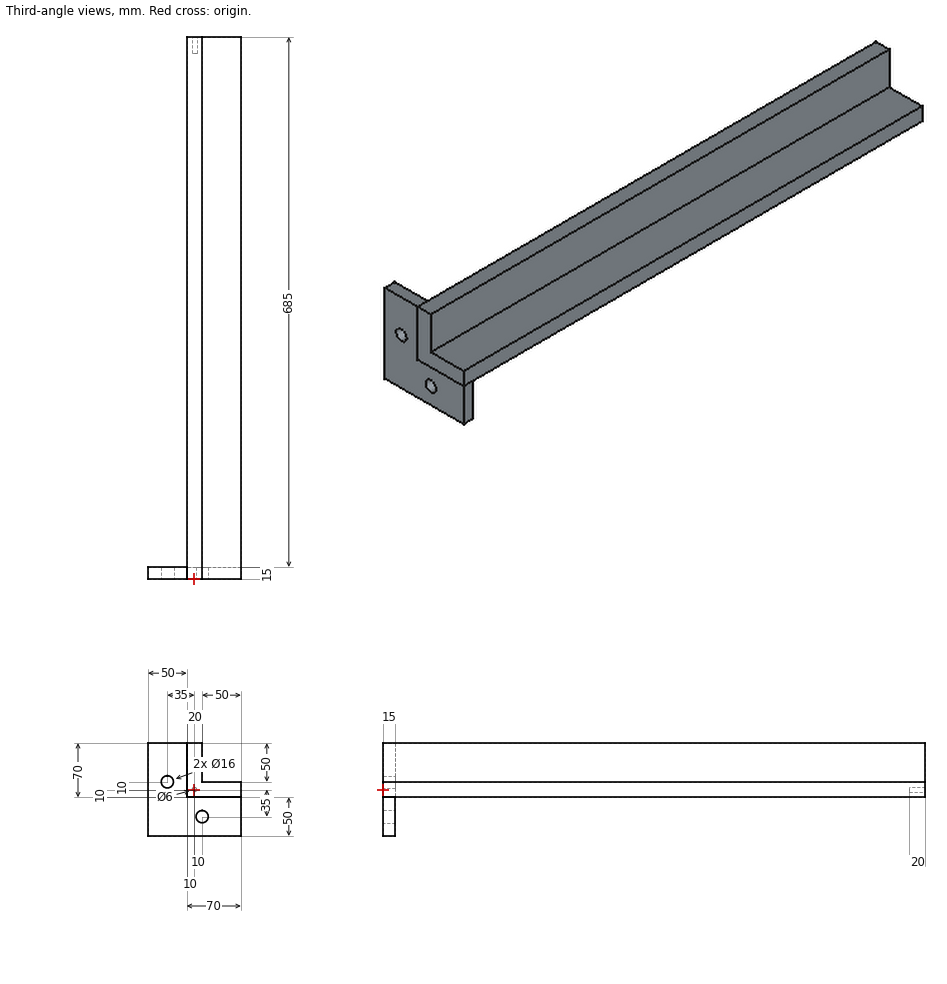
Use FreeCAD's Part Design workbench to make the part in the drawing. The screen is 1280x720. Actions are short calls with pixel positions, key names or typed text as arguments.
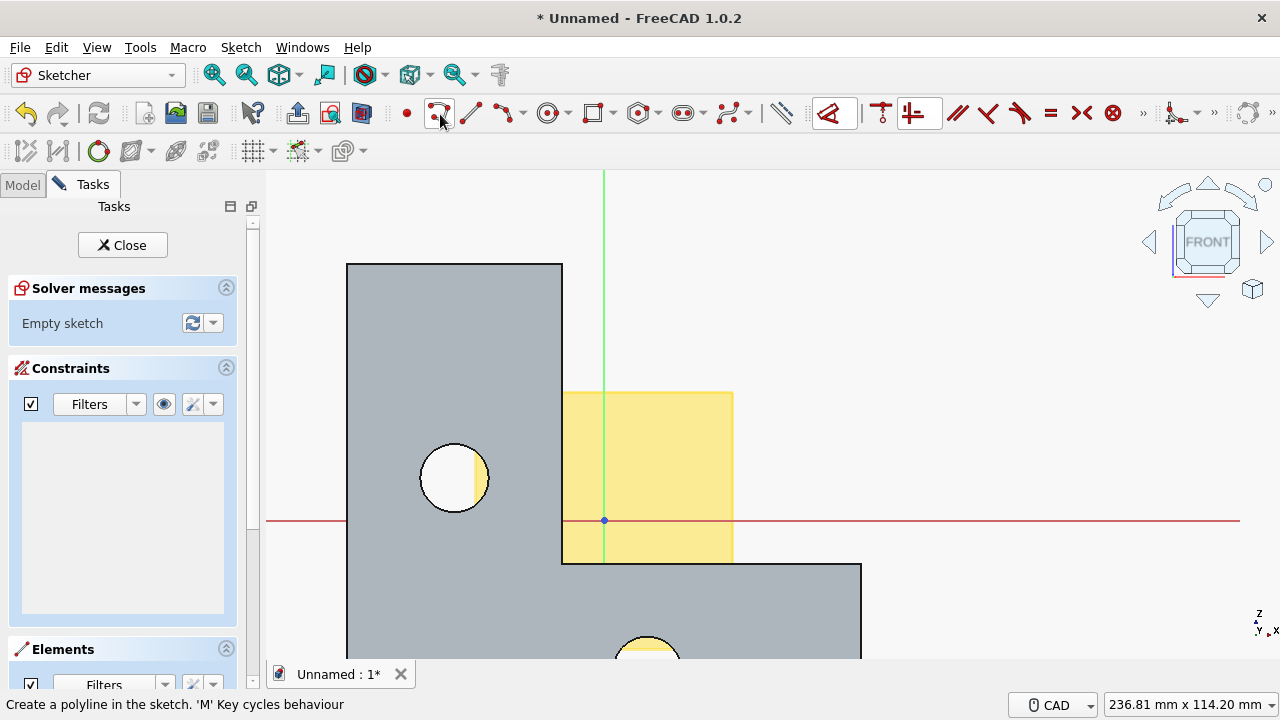
click(562, 564)
click(562, 264)
click(647, 264)
click(647, 478)
click(861, 478)
click(861, 564)
click(562, 565)
key(Escape)
key(Escape)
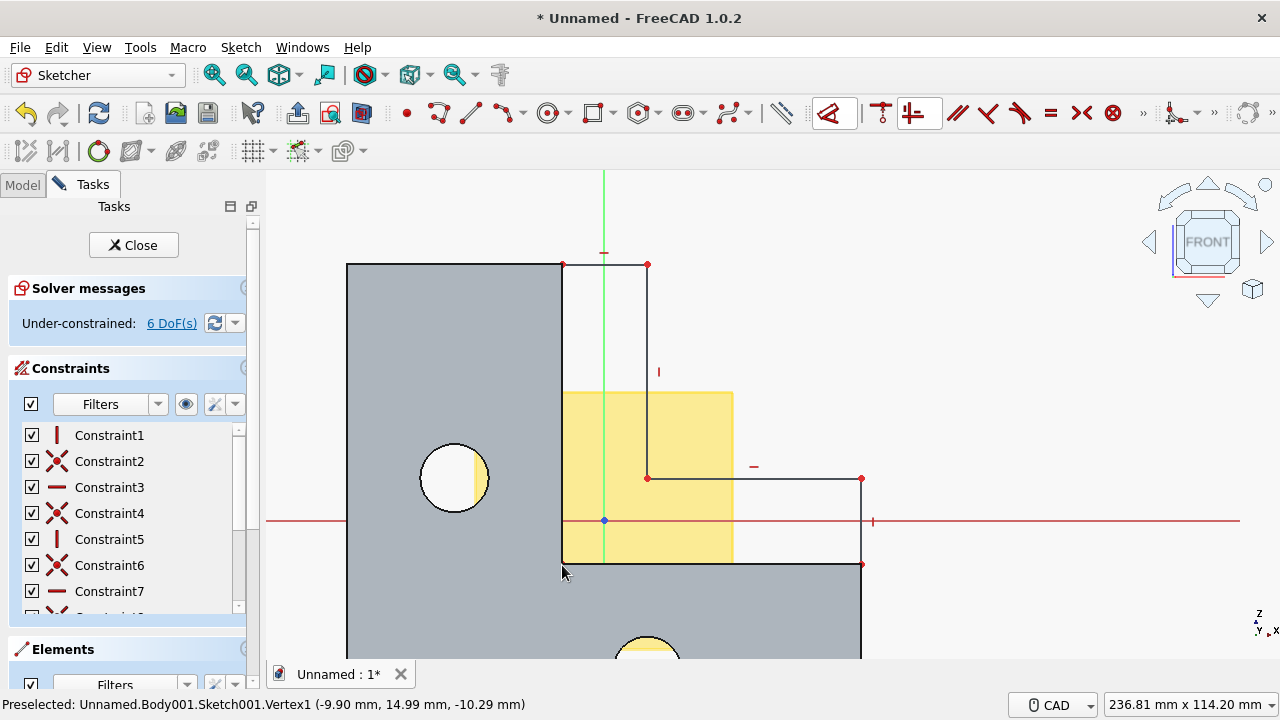
click(562, 475)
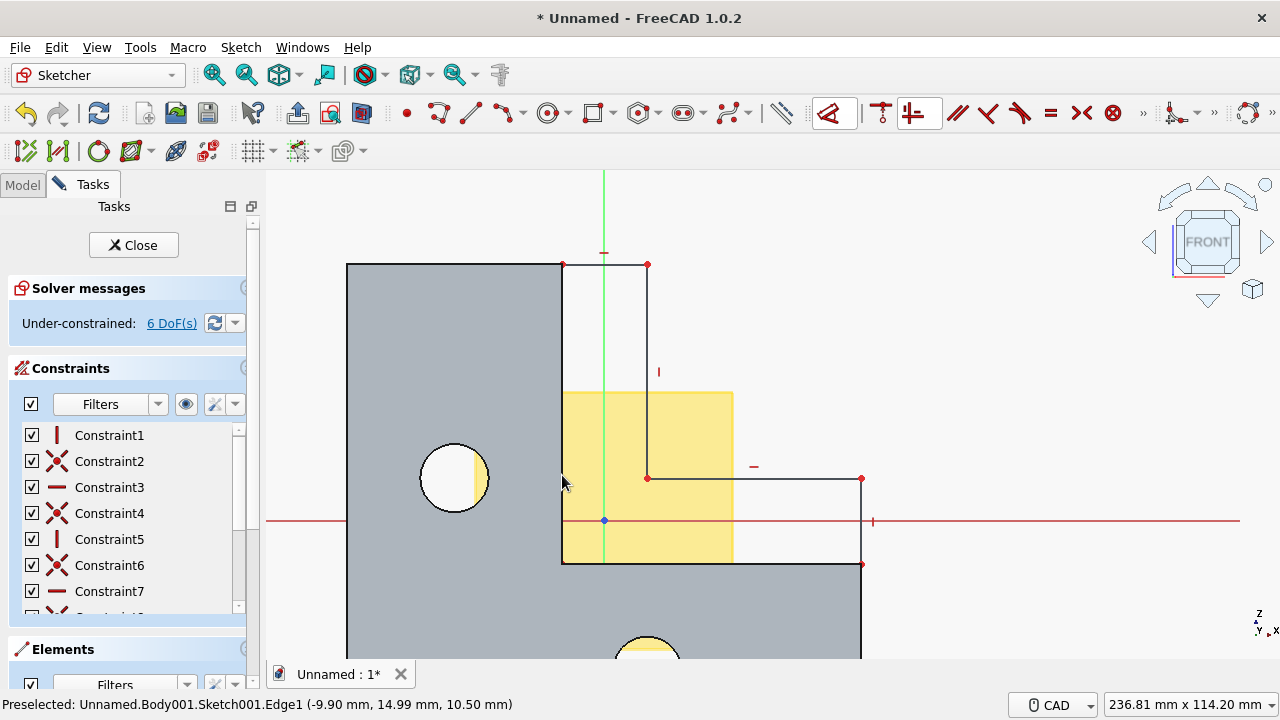
key(i)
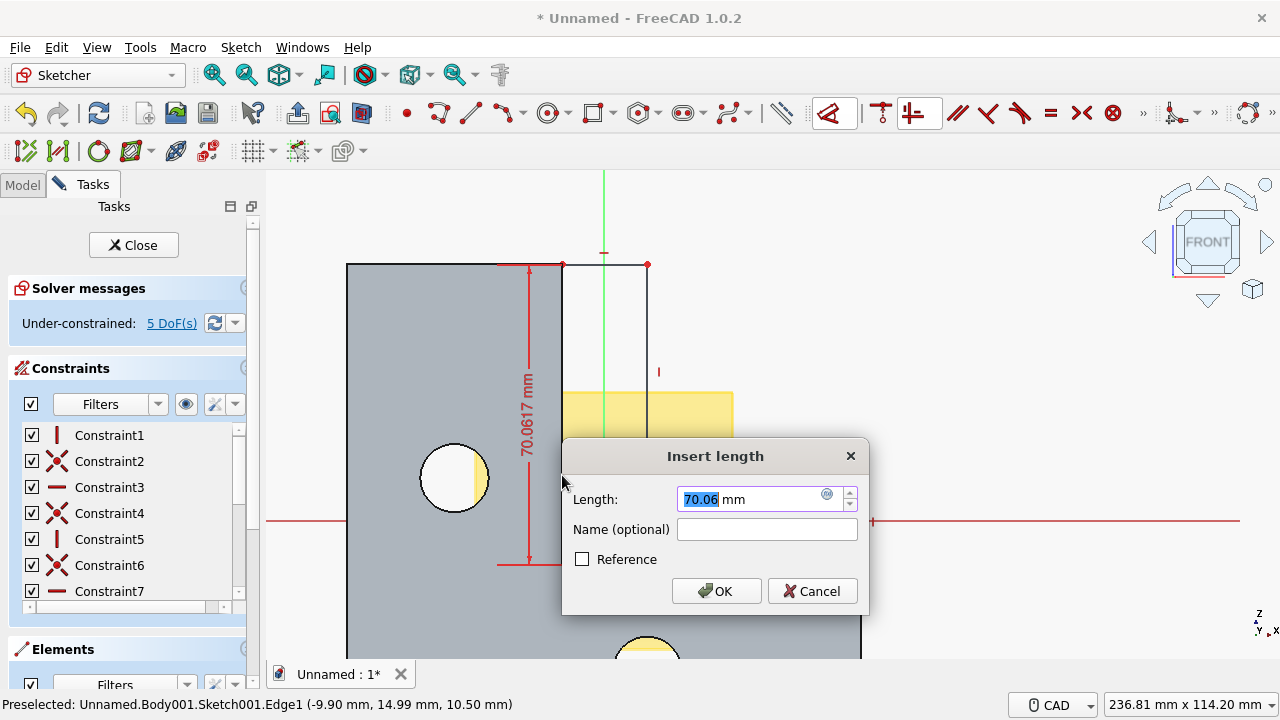
text(70)
key(Return)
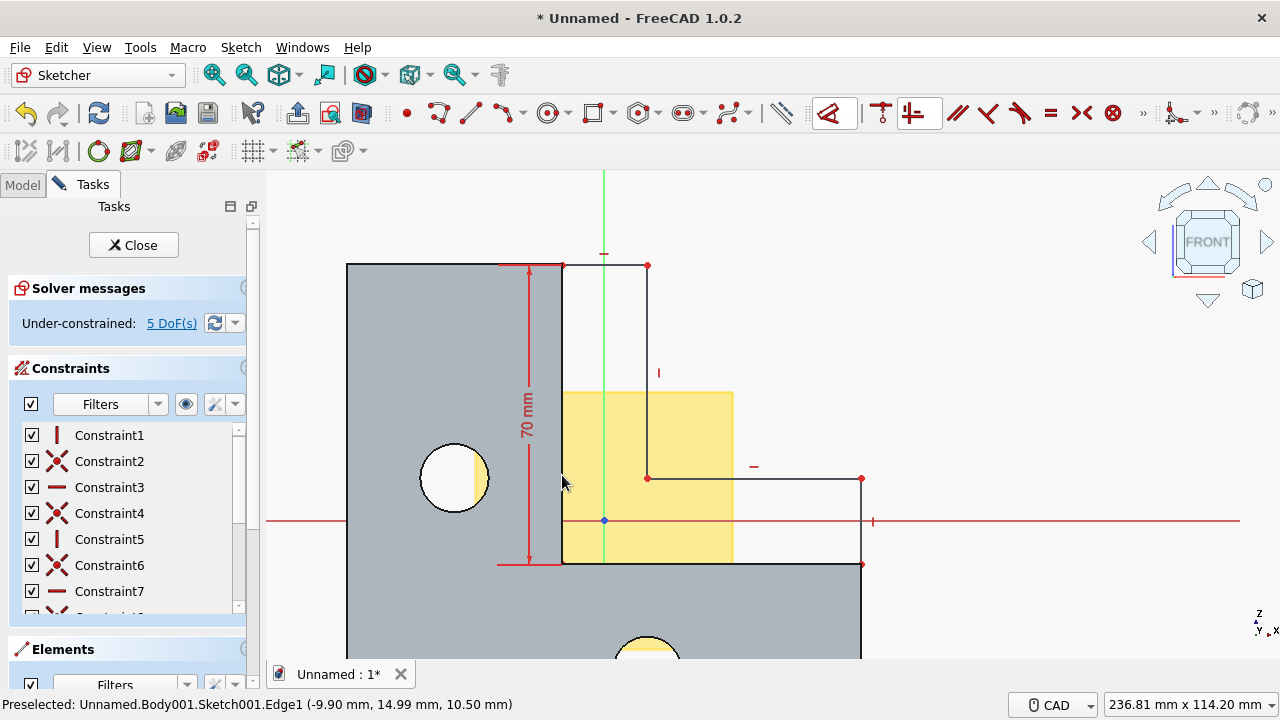
click(588, 265)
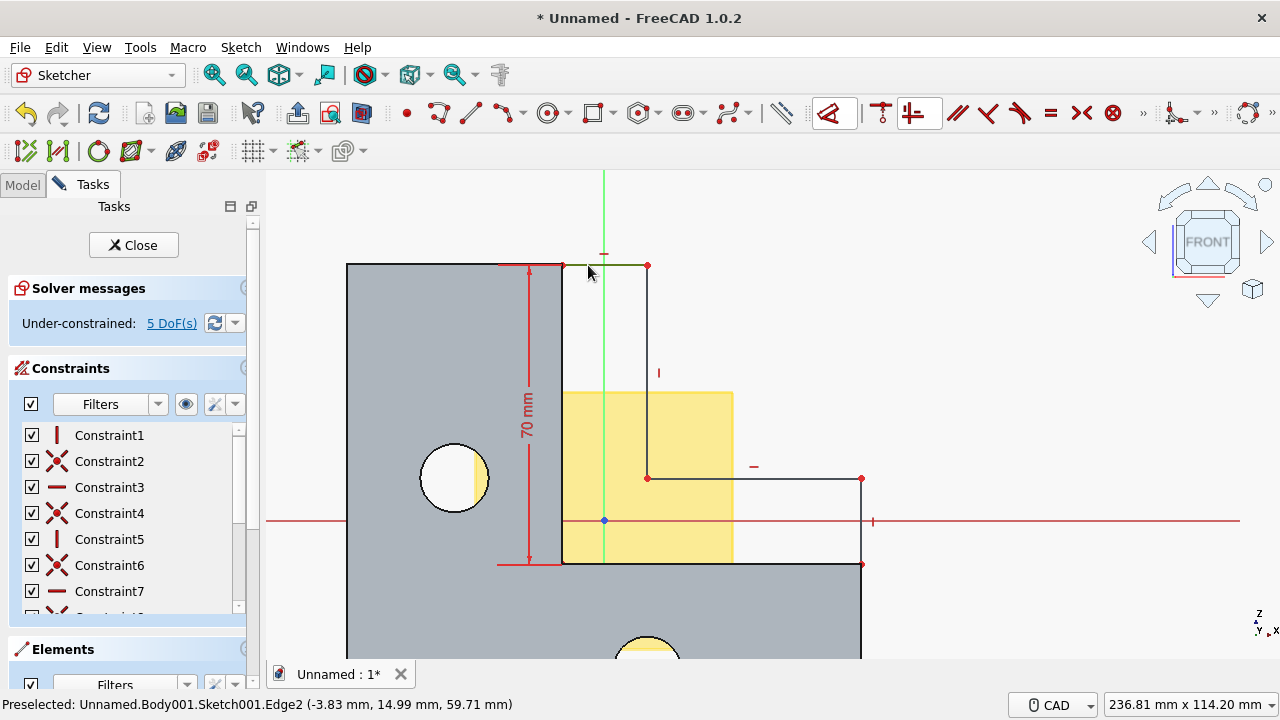
click(852, 114)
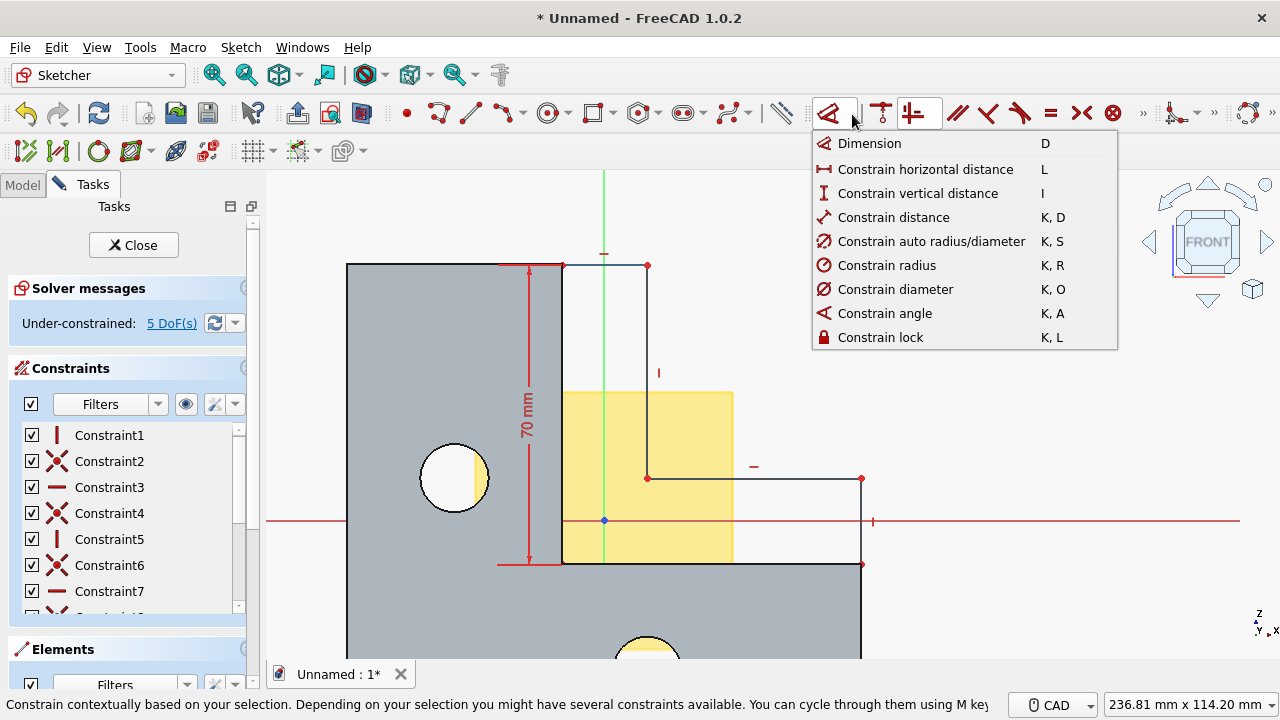
click(965, 169)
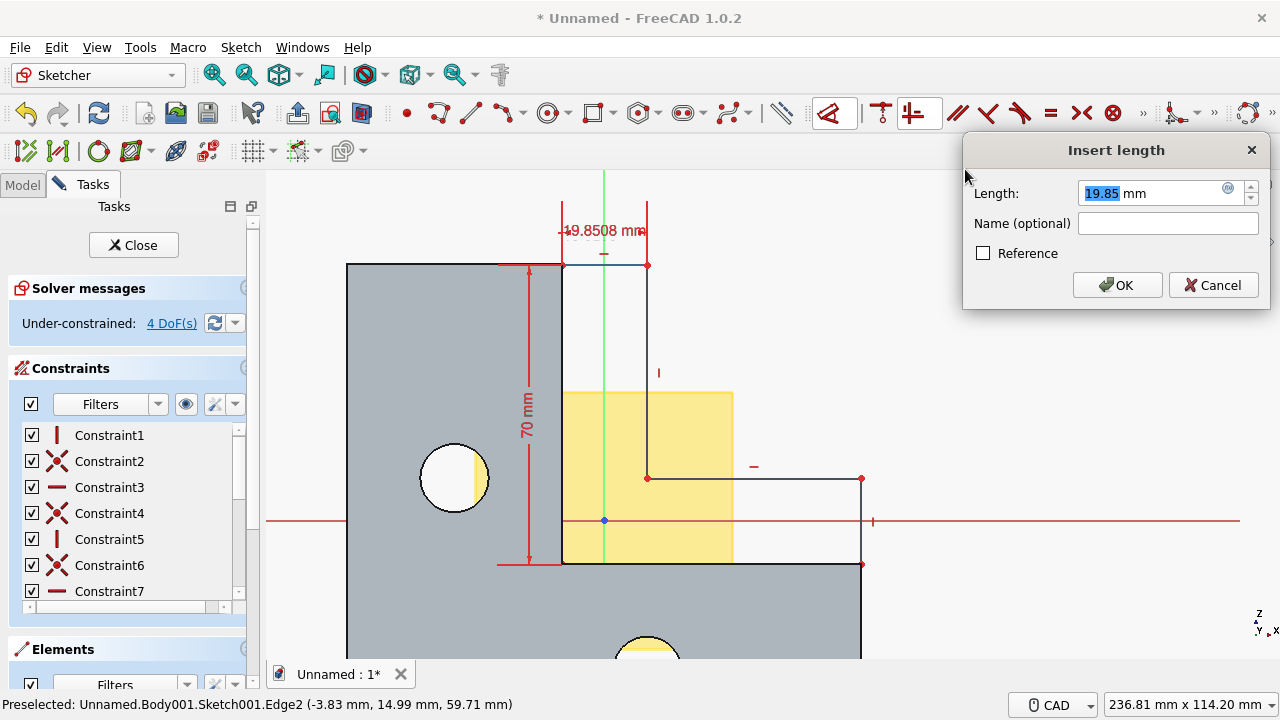
text(20)
key(Return)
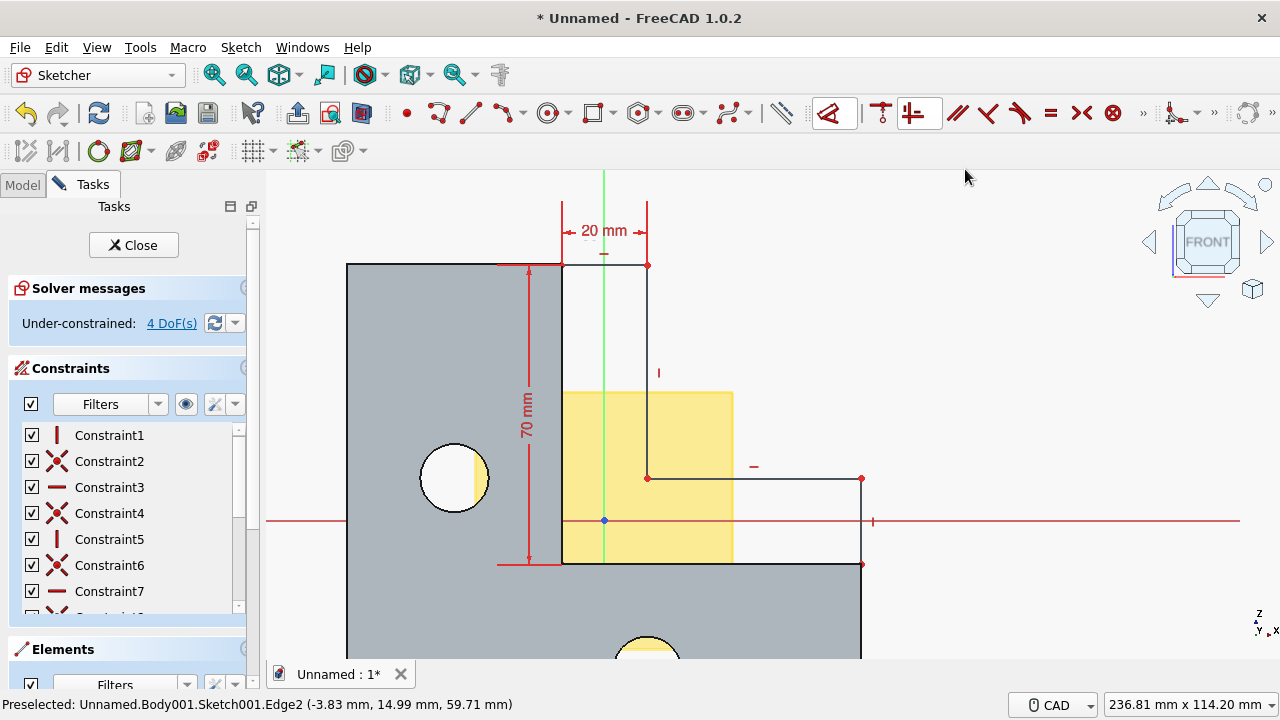
click(647, 329)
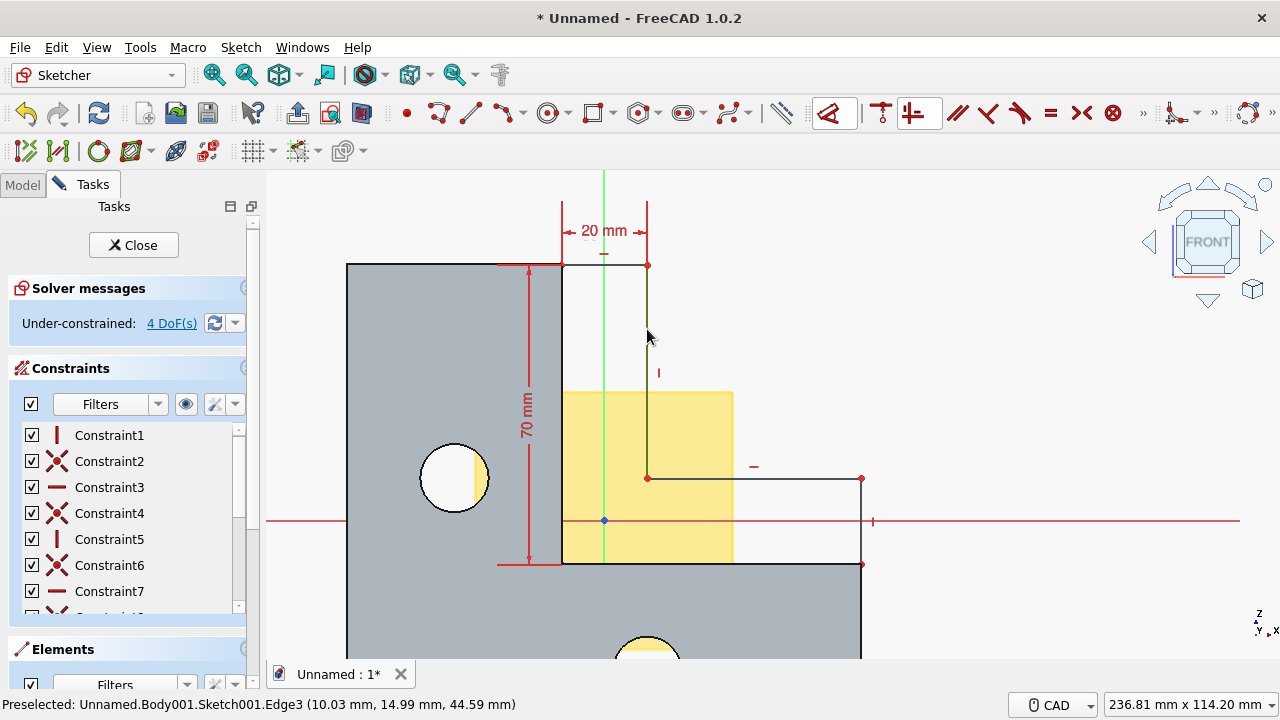
key(i)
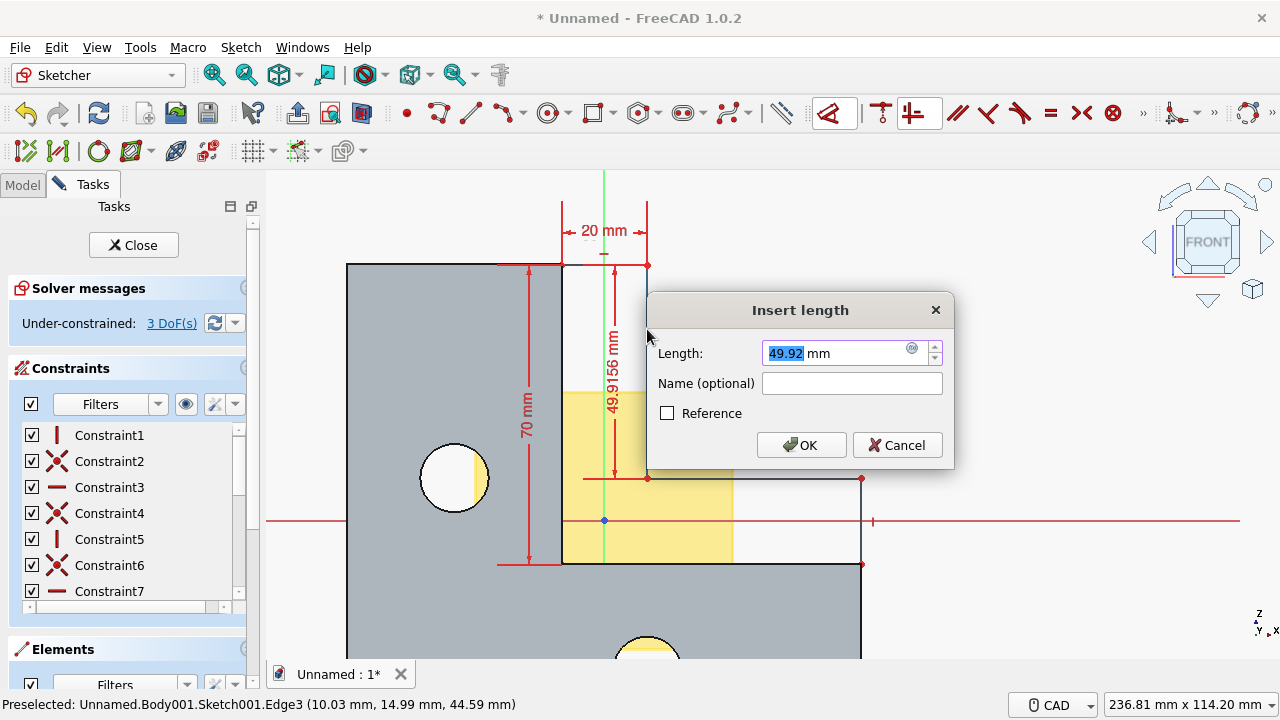
text(50)
key(Return)